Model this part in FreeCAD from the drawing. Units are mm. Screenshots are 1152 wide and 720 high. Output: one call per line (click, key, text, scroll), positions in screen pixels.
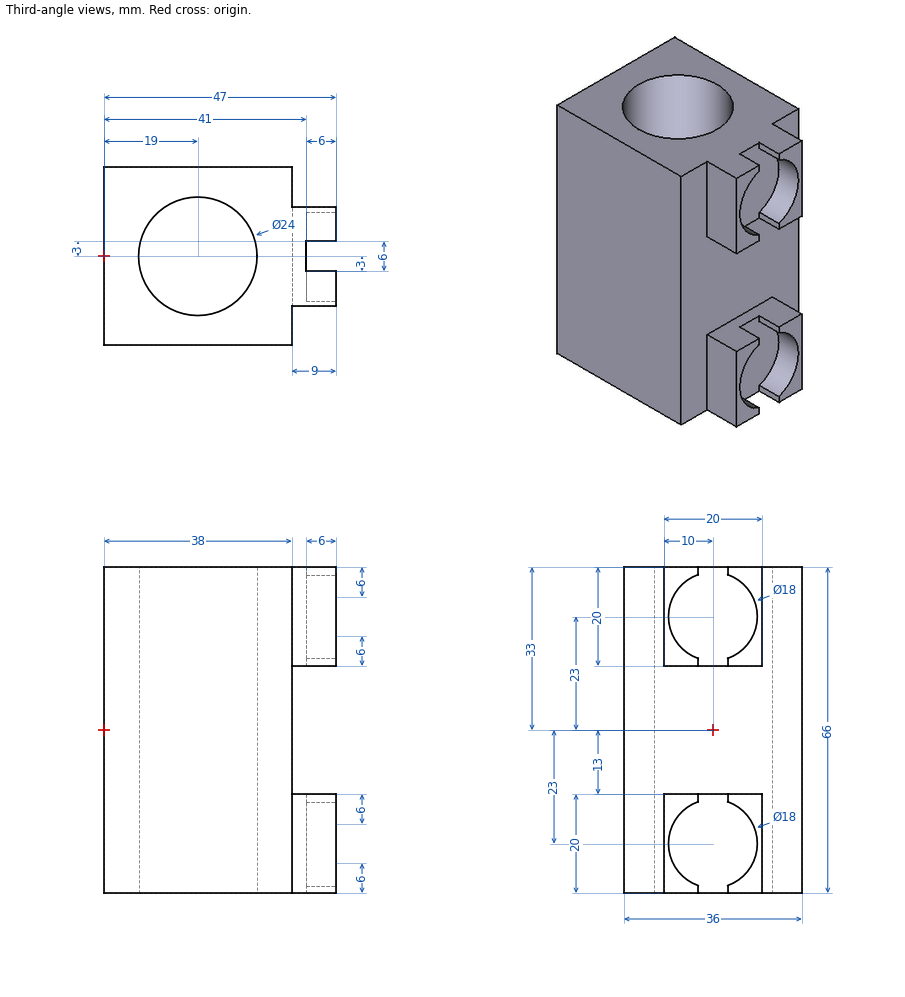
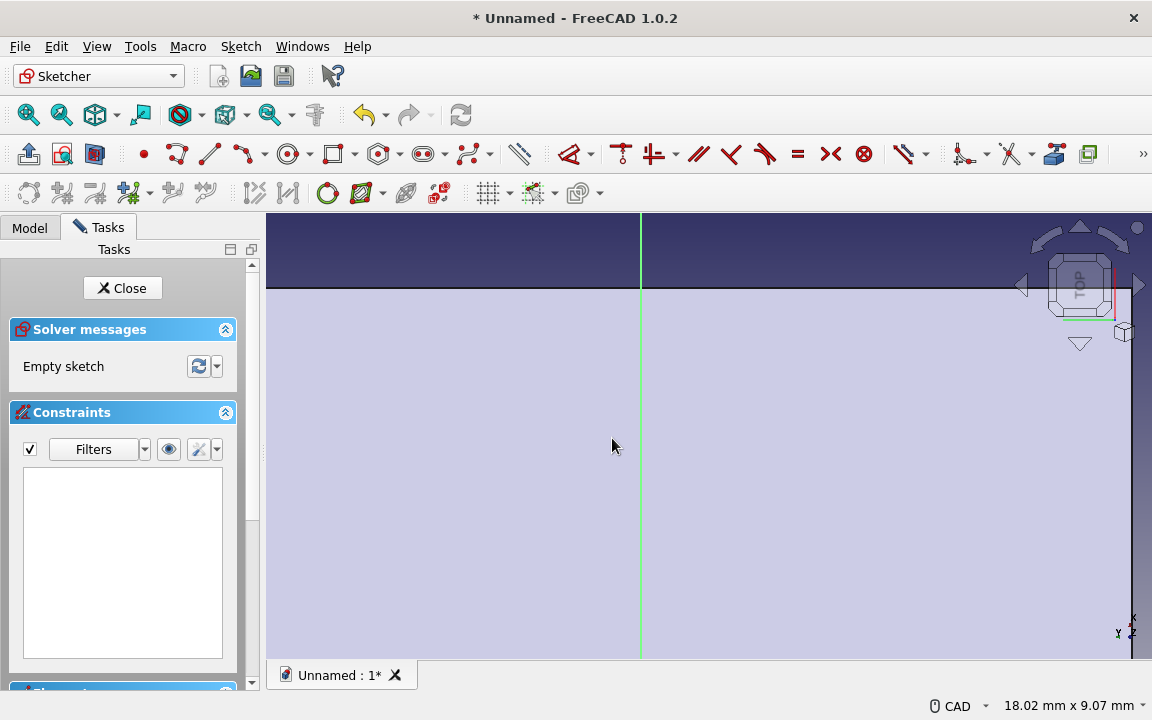
click(332, 154)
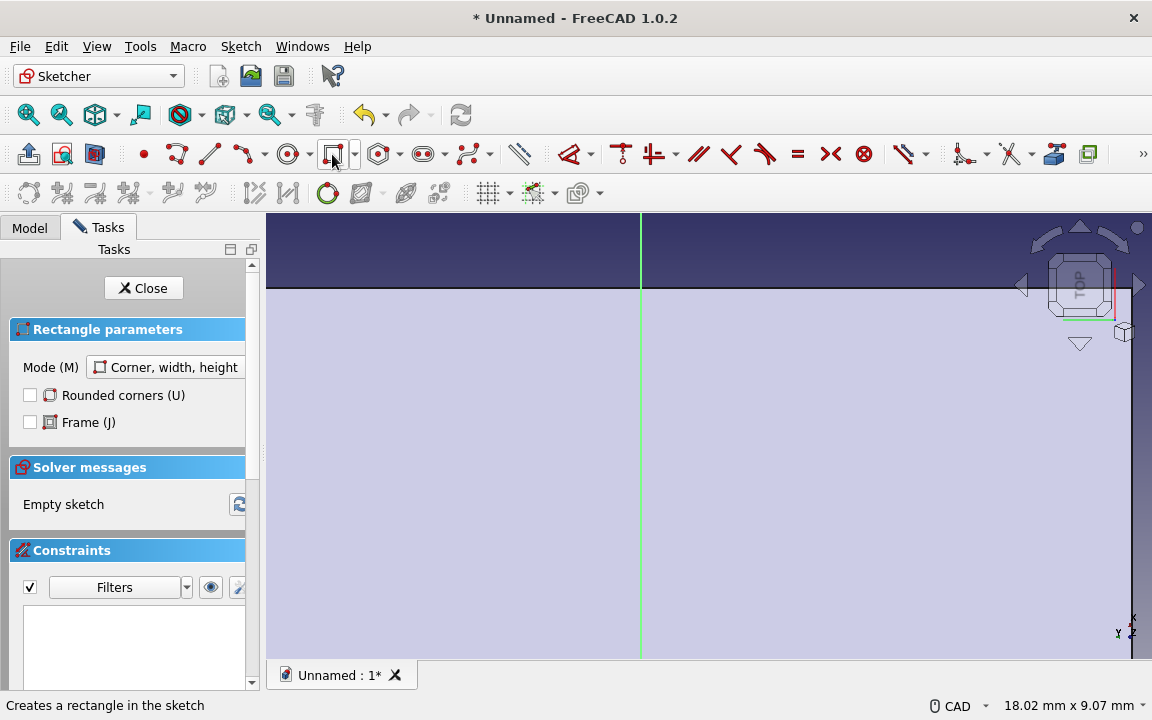
click(493, 288)
click(788, 583)
key(Escape)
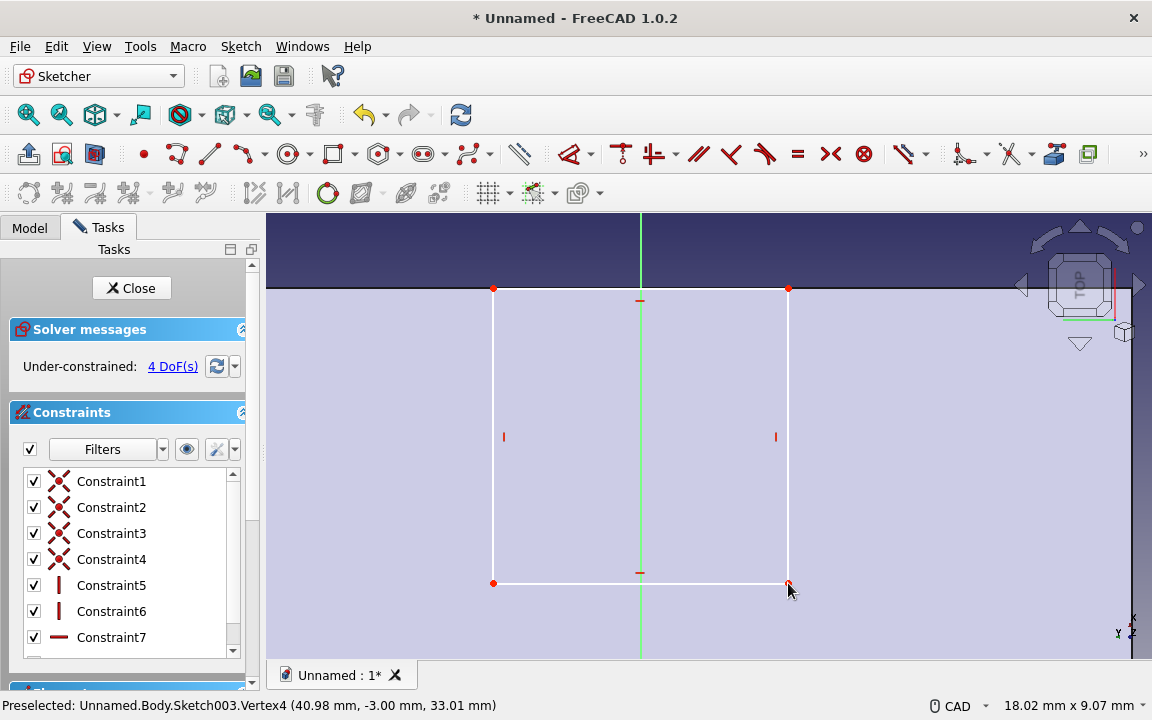
click(568, 154)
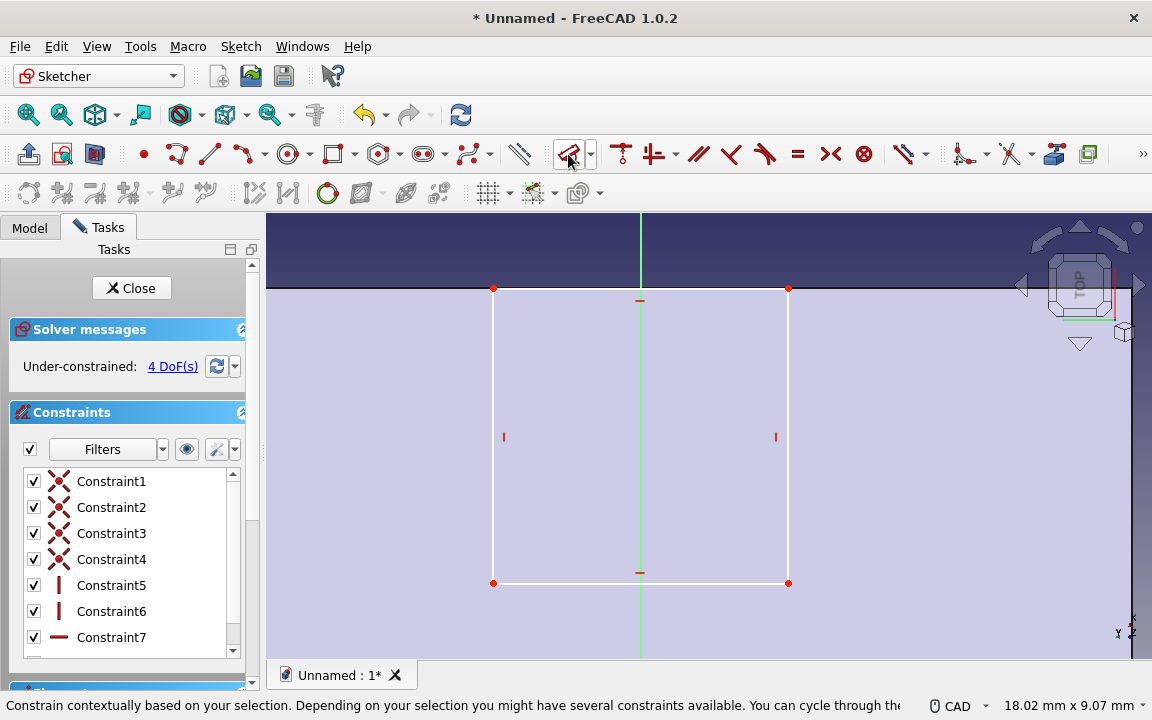
click(493, 378)
click(459, 437)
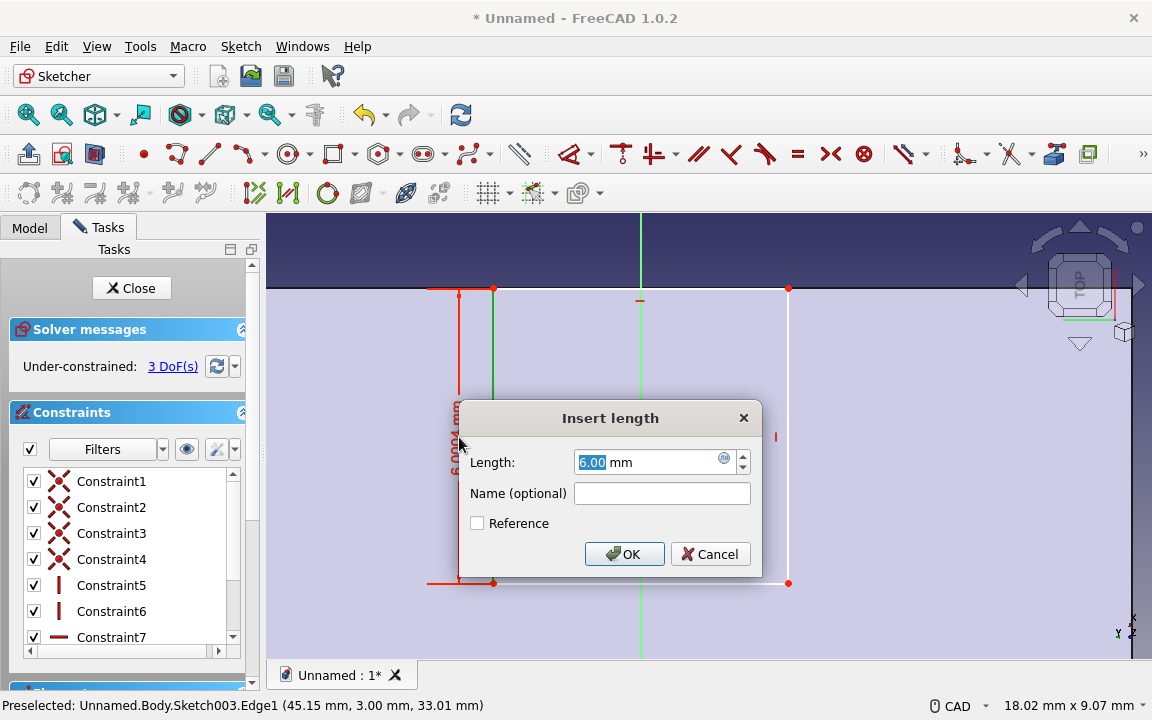
text(6)
key(Return)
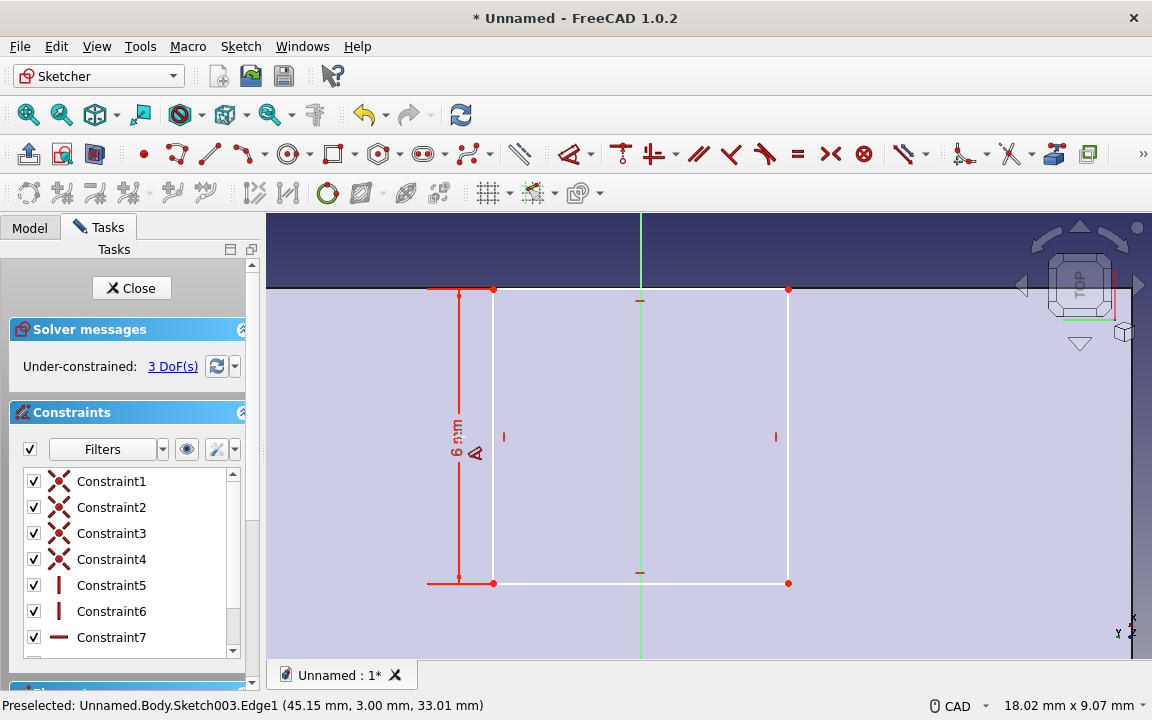
click(582, 584)
click(573, 618)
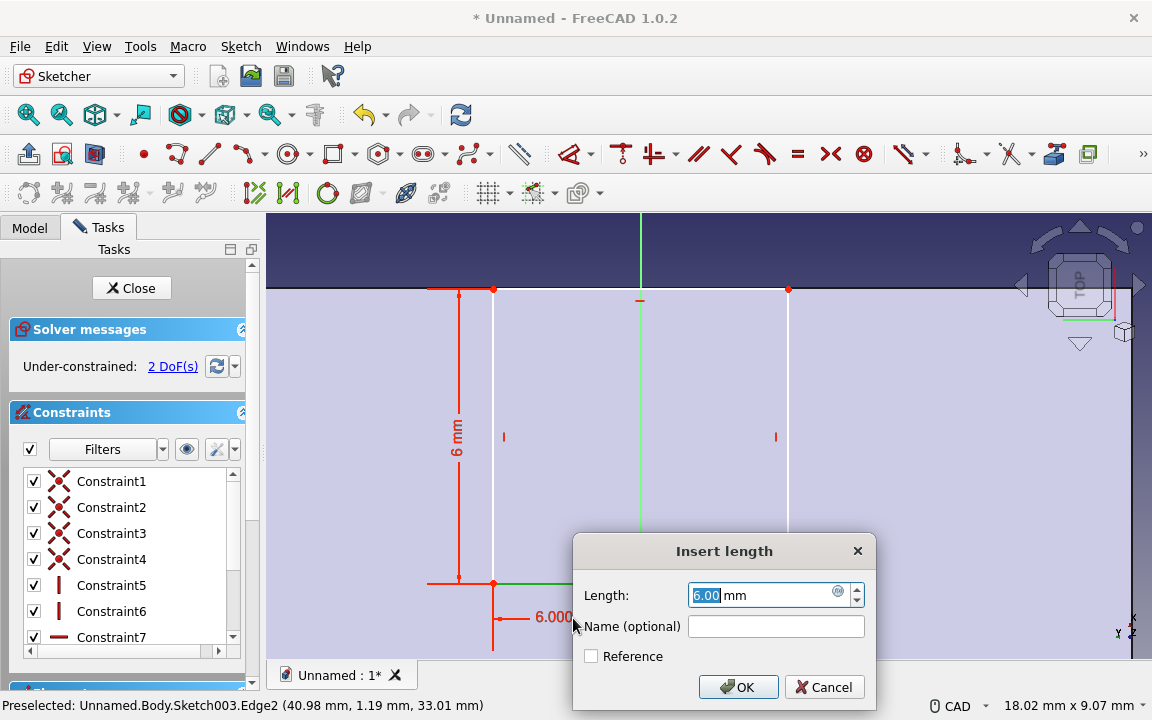
text(6)
key(Return)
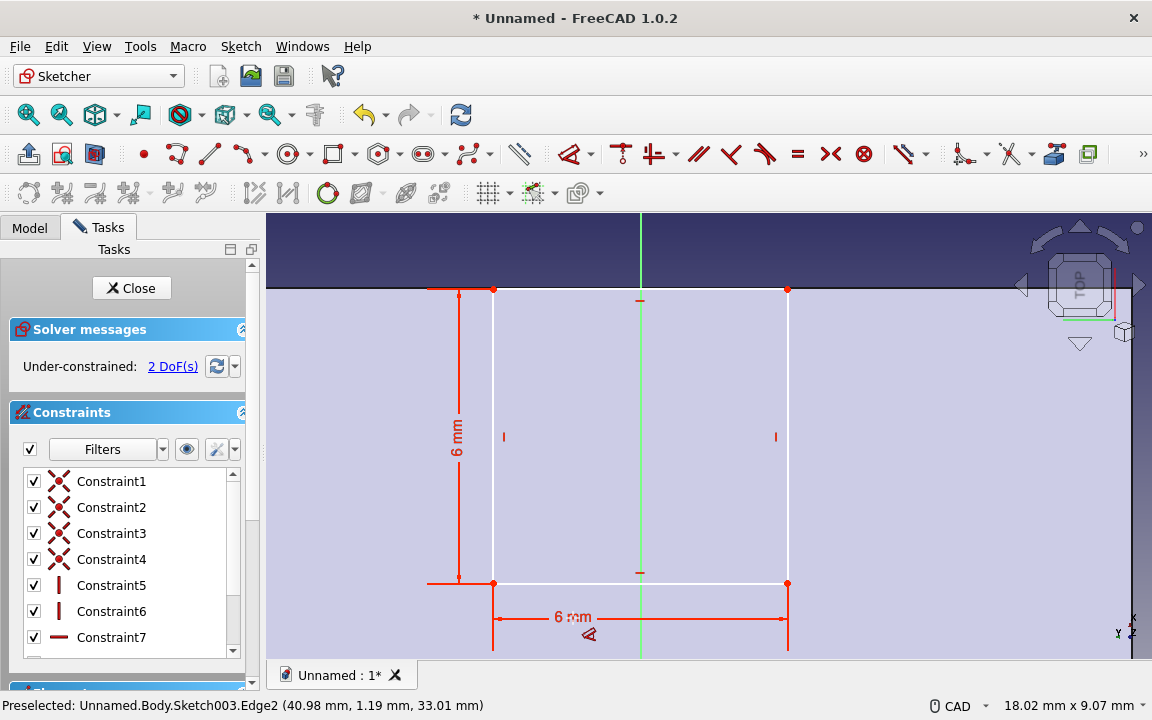
click(493, 289)
click(567, 255)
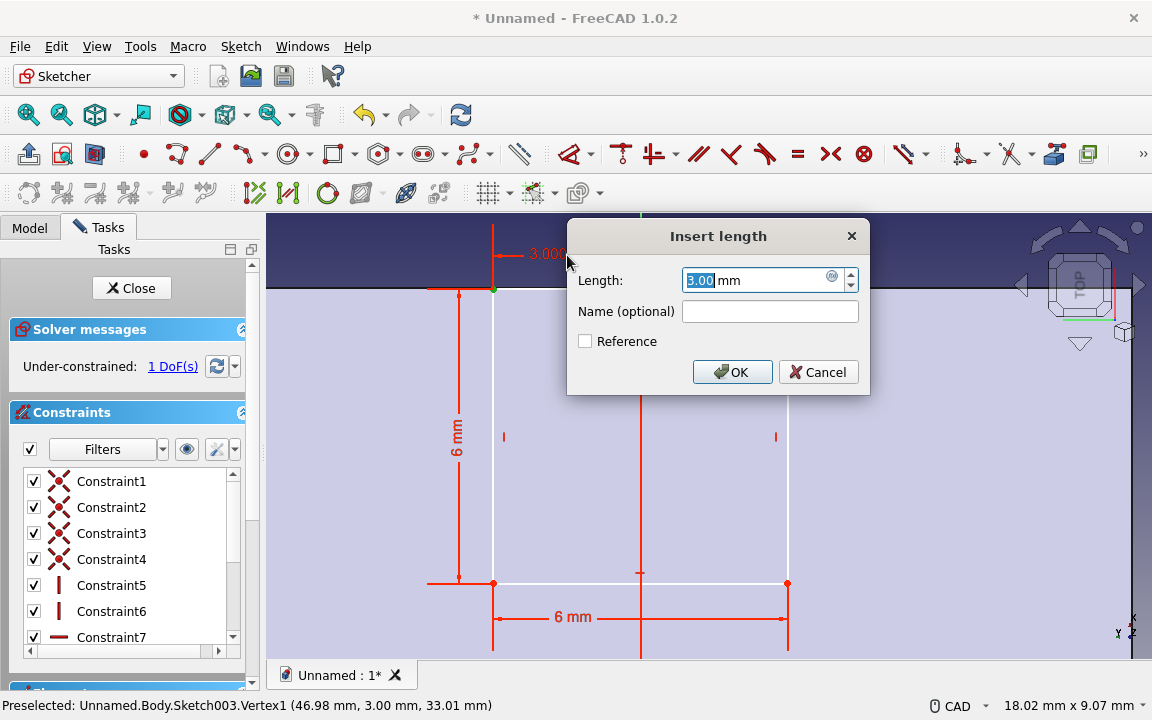
text(3)
key(Return)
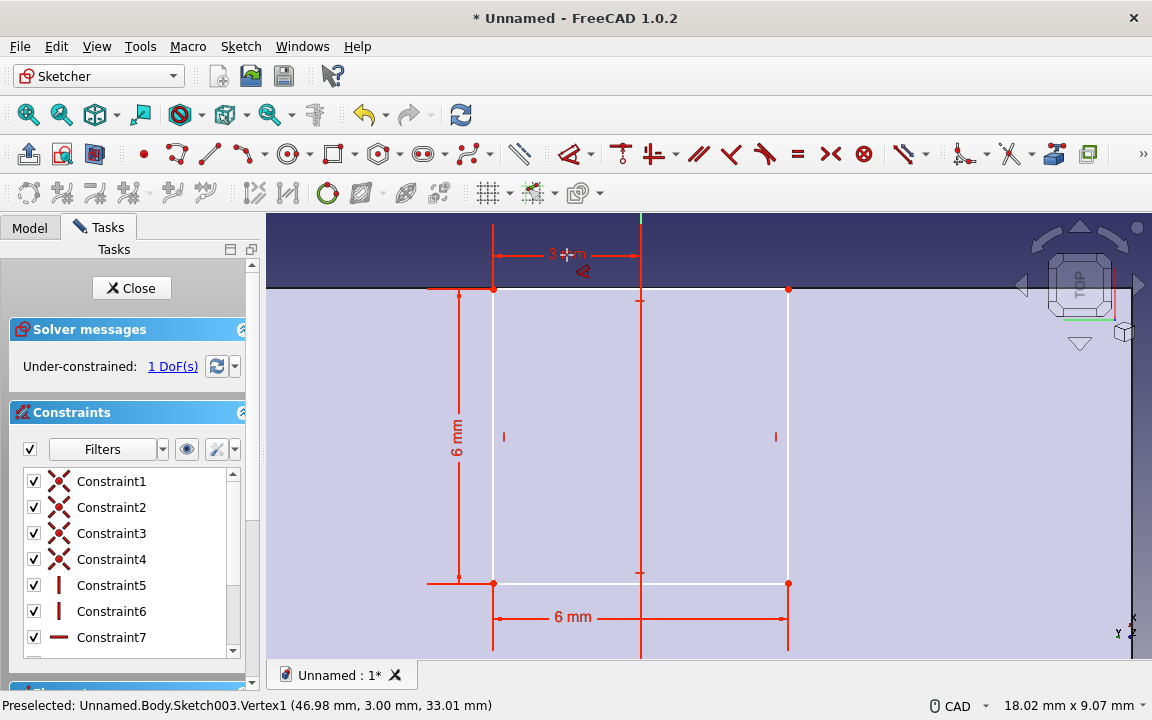
click(493, 289)
click(459, 460)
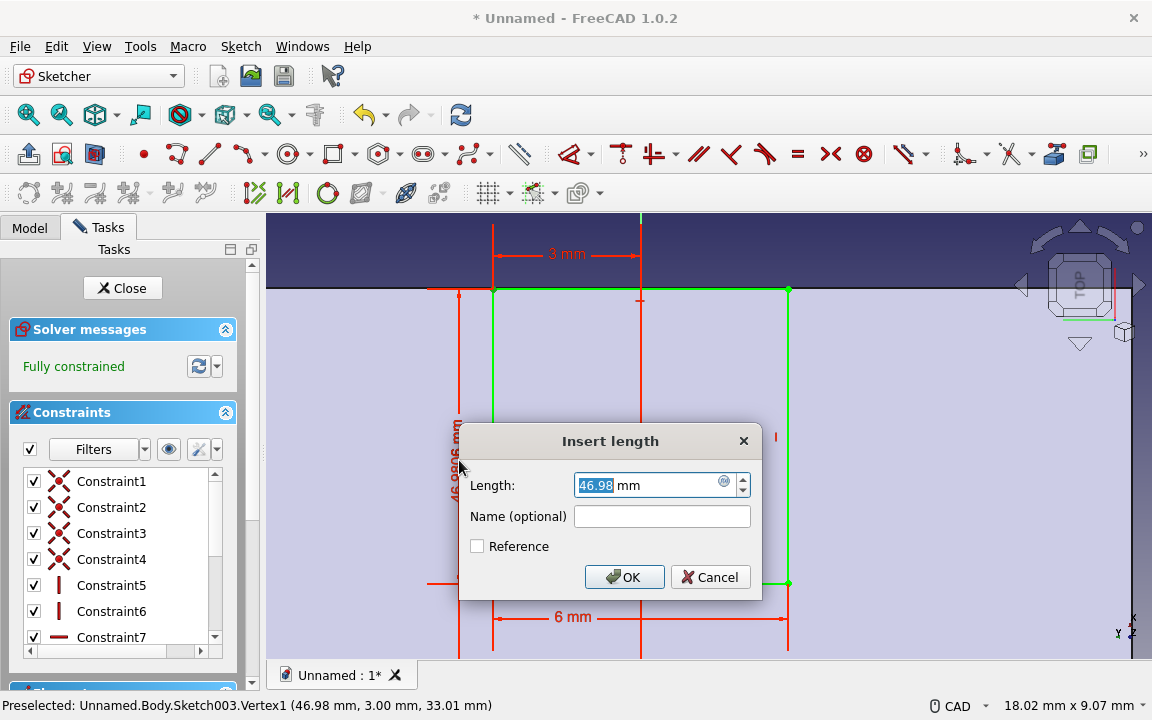
text(47)
key(Return)
key(Escape)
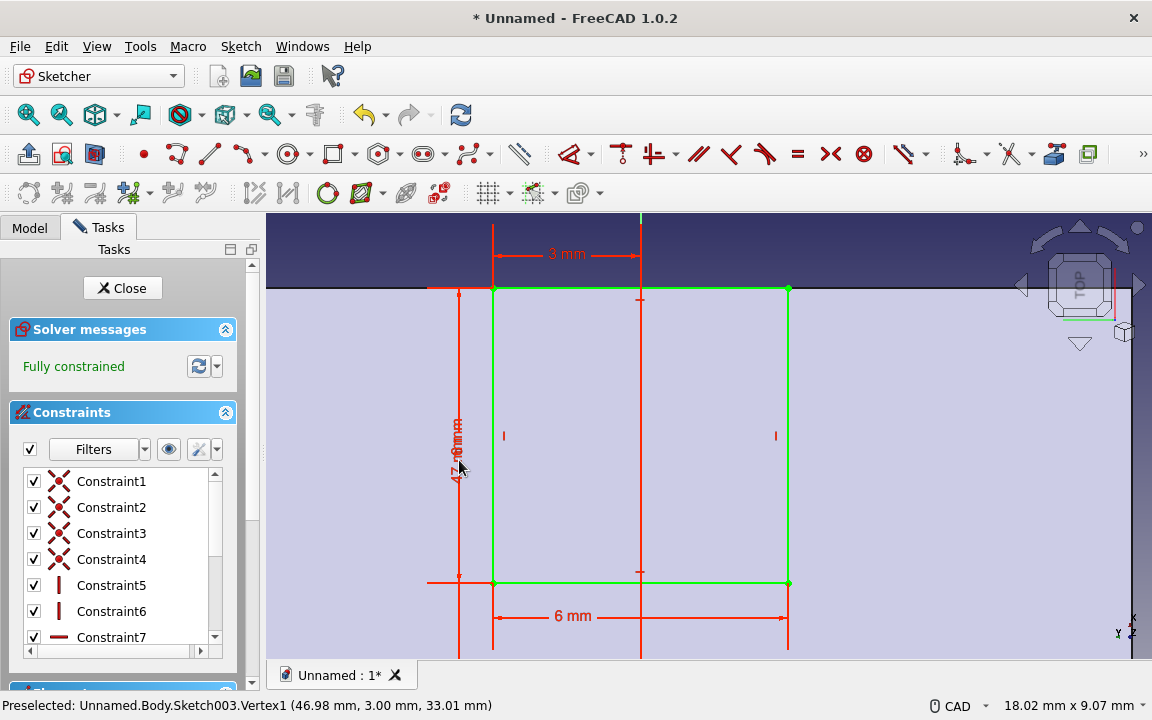
click(123, 288)